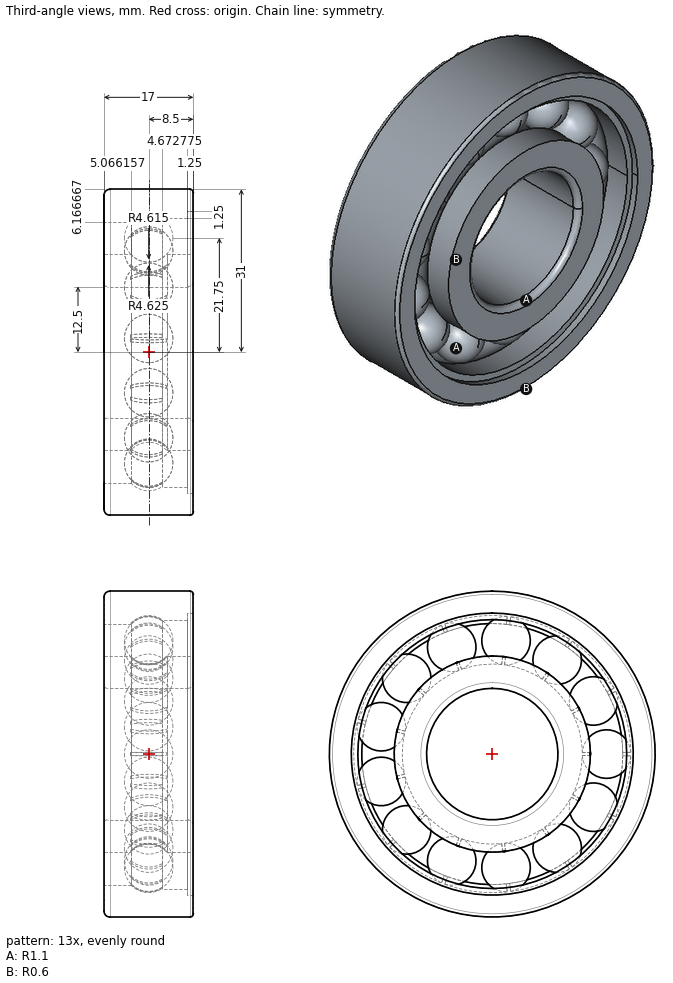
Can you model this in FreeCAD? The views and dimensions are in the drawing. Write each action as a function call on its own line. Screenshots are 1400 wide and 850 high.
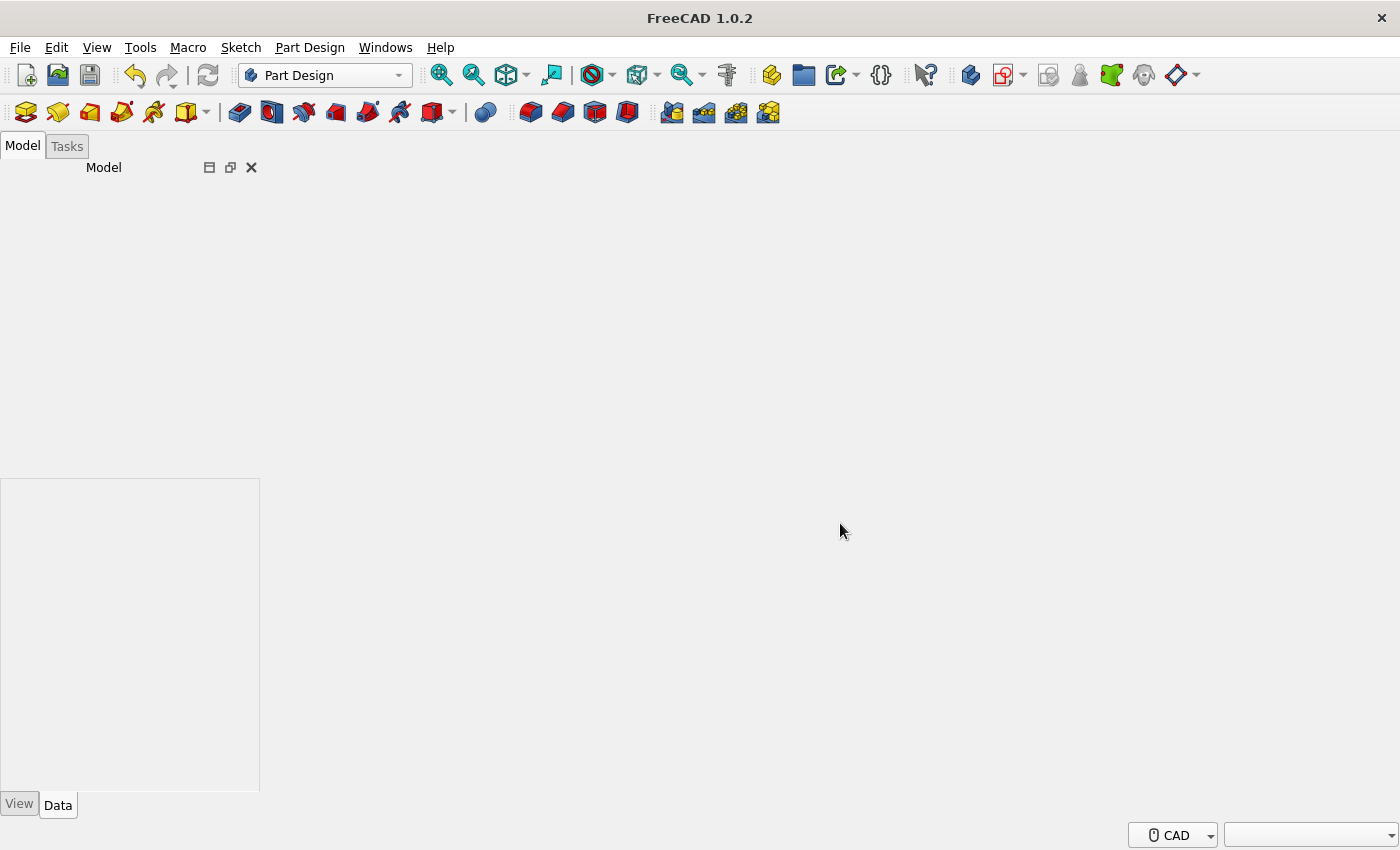
click(26, 76)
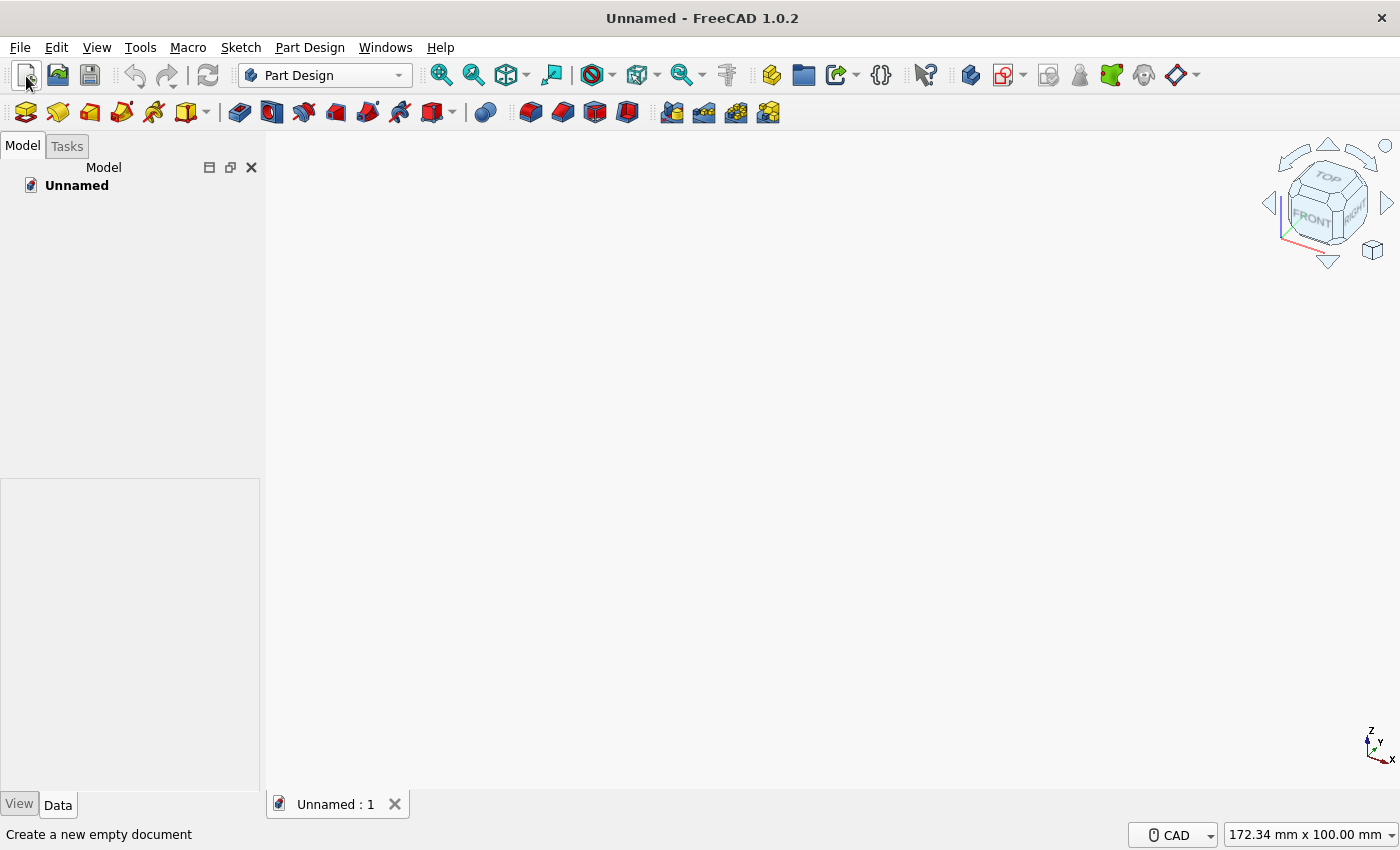
click(1004, 76)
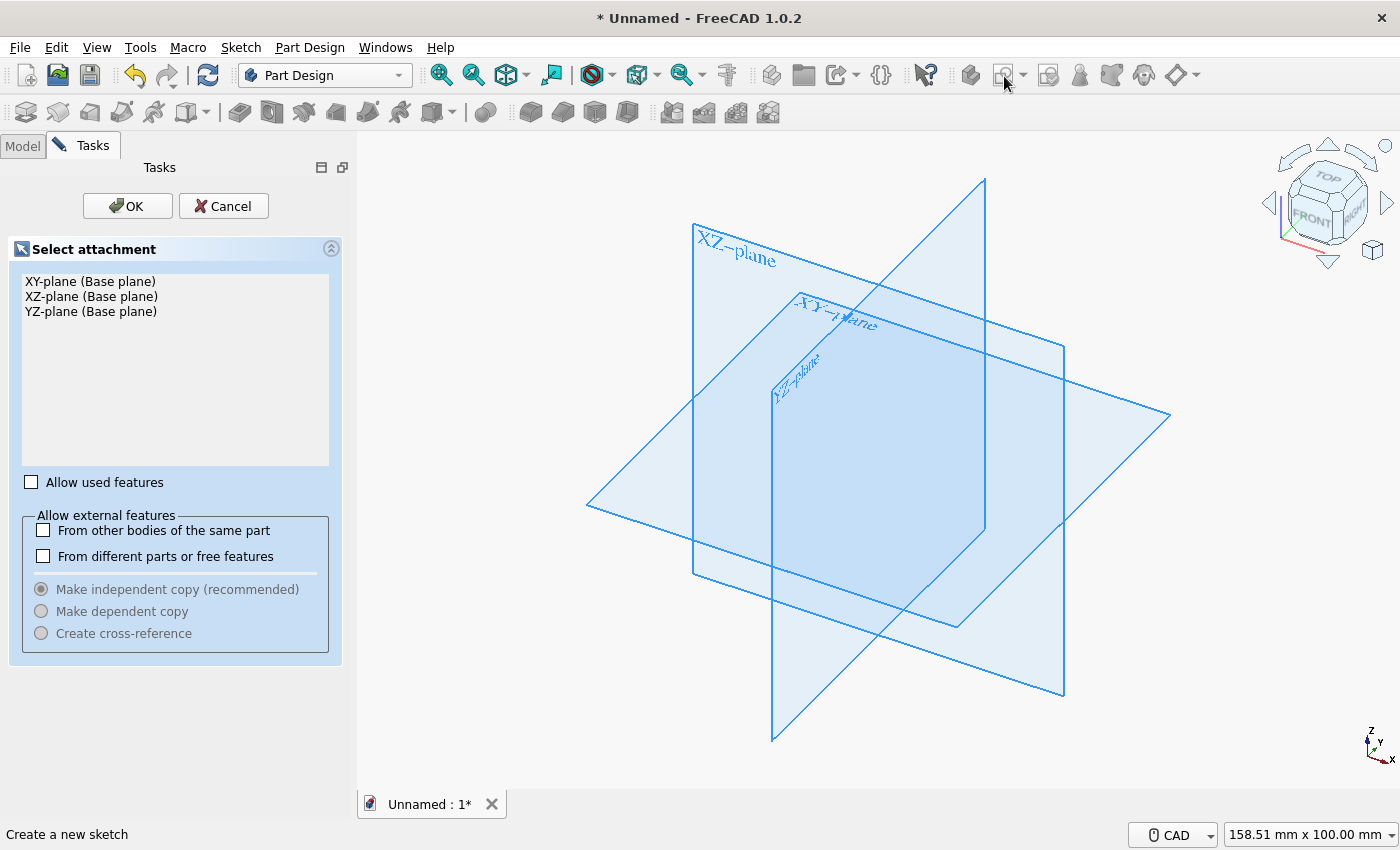
click(82, 282)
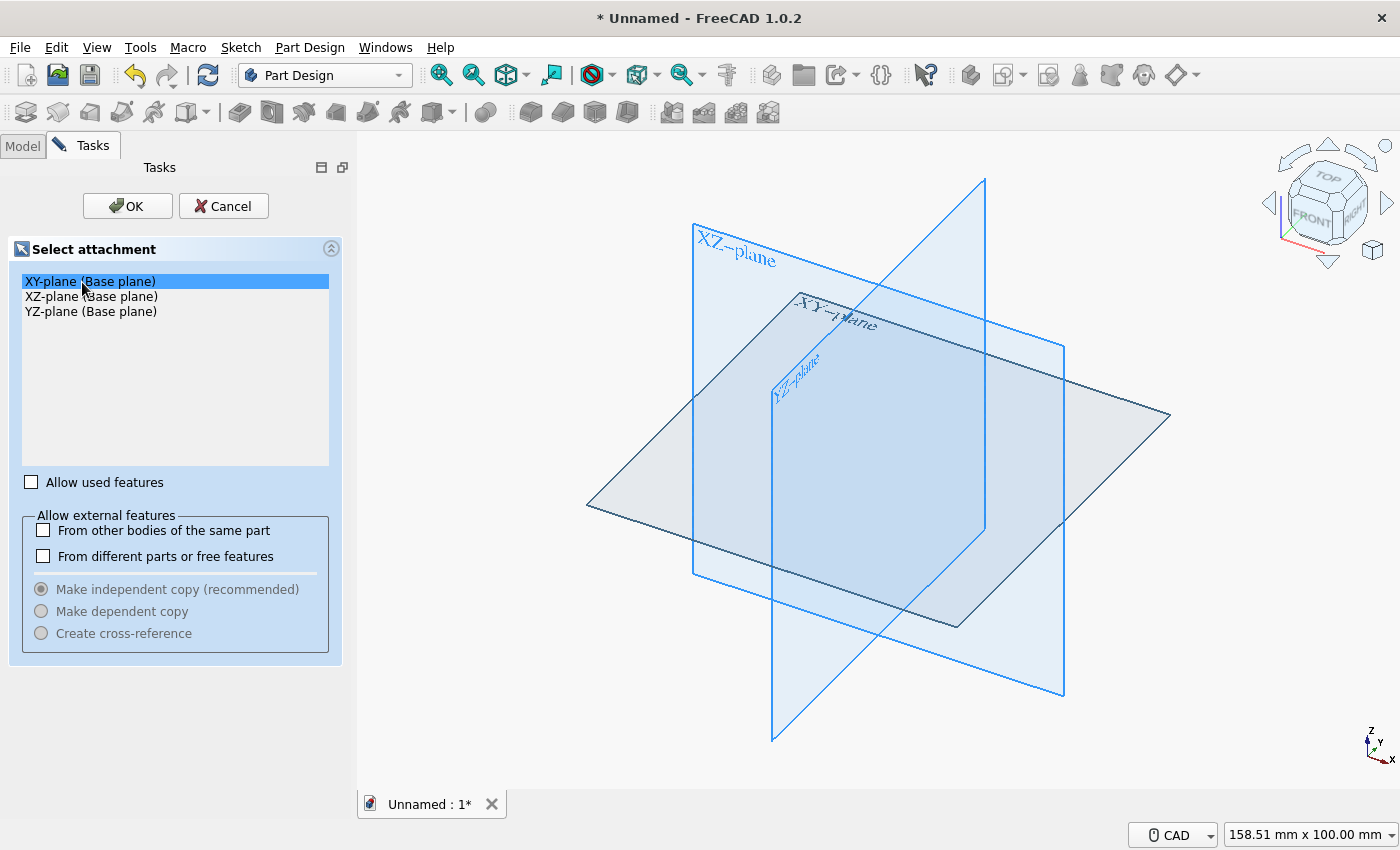
click(128, 206)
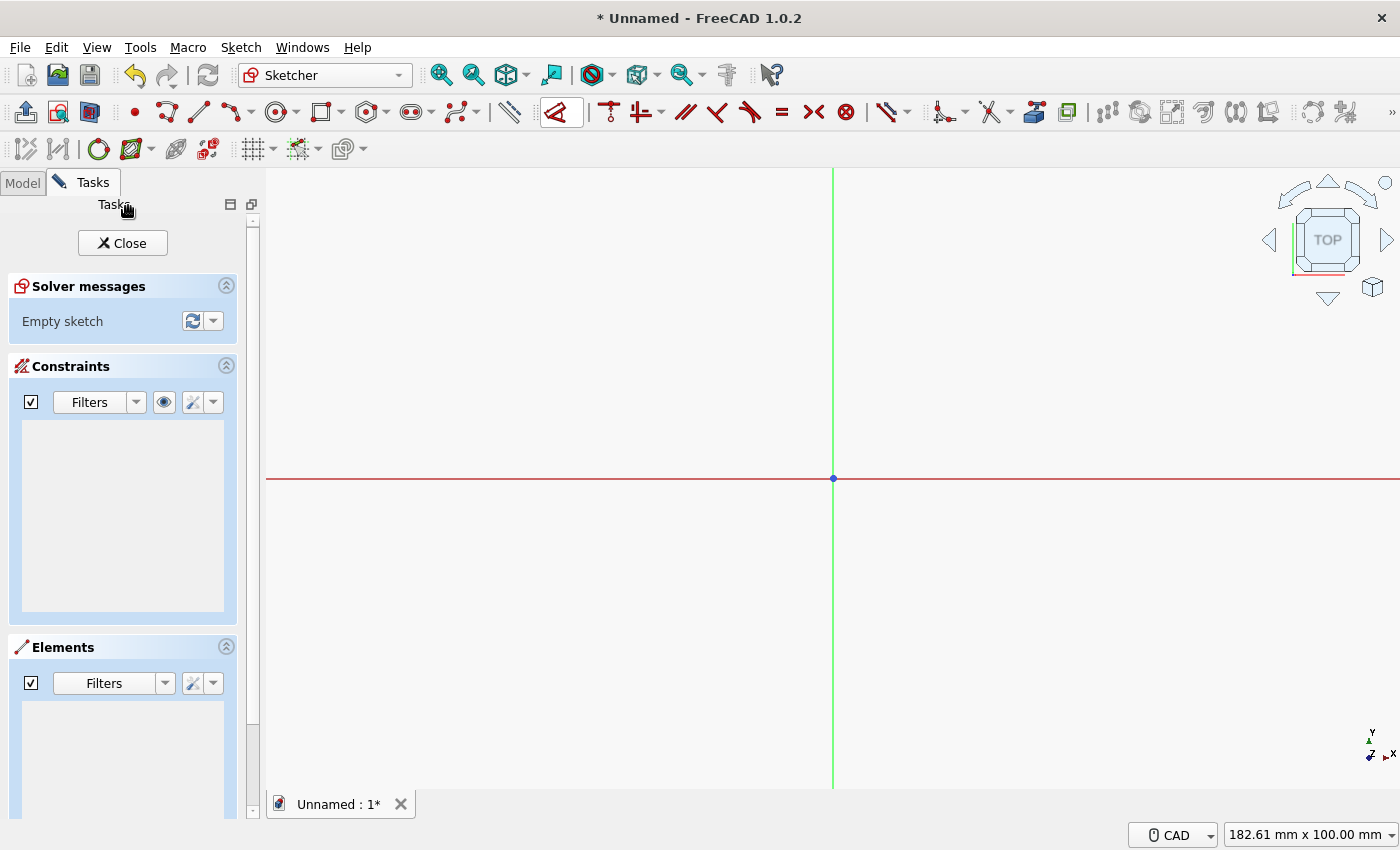
scroll(891, 372, up, 5)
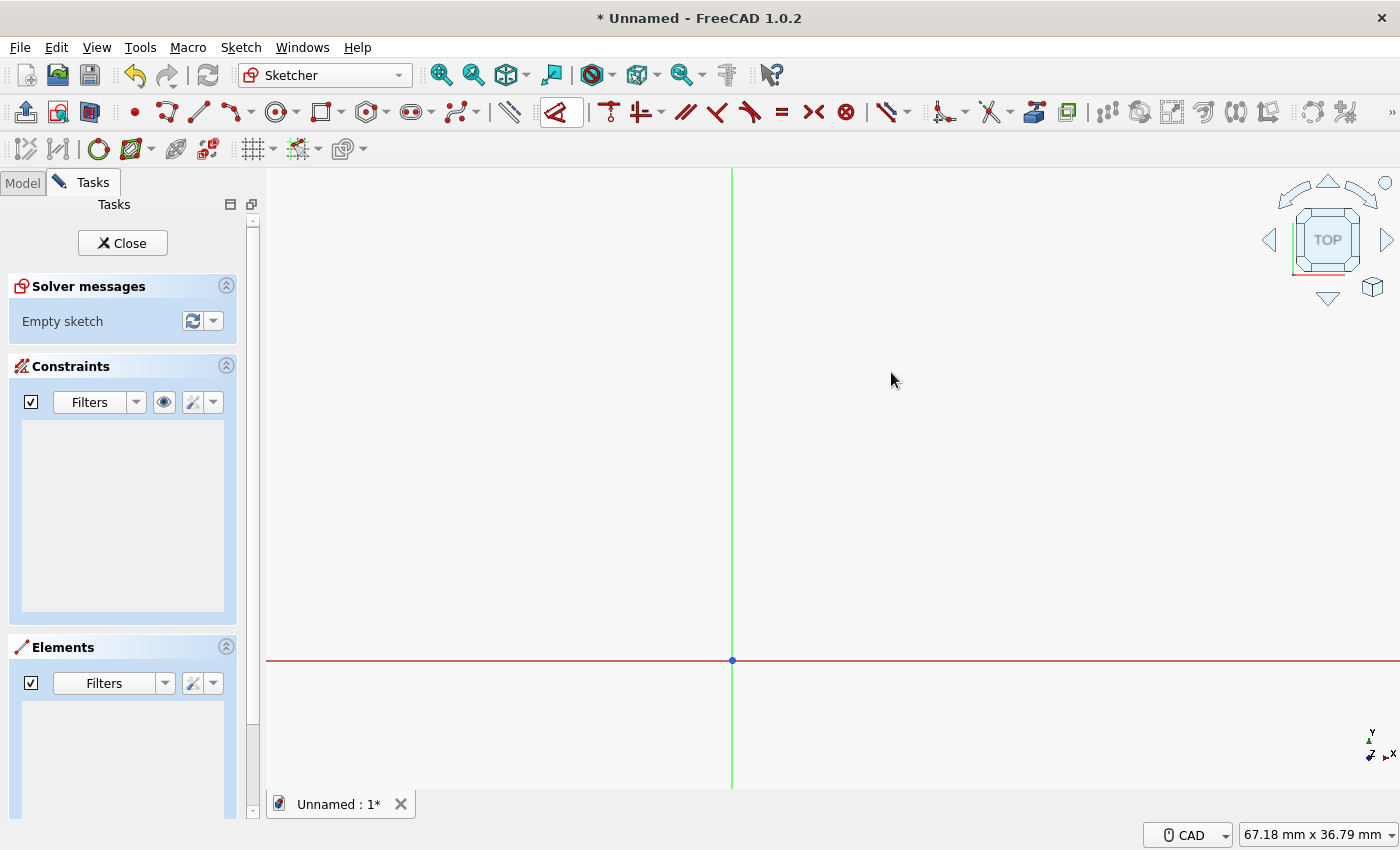
key(g)
key(l)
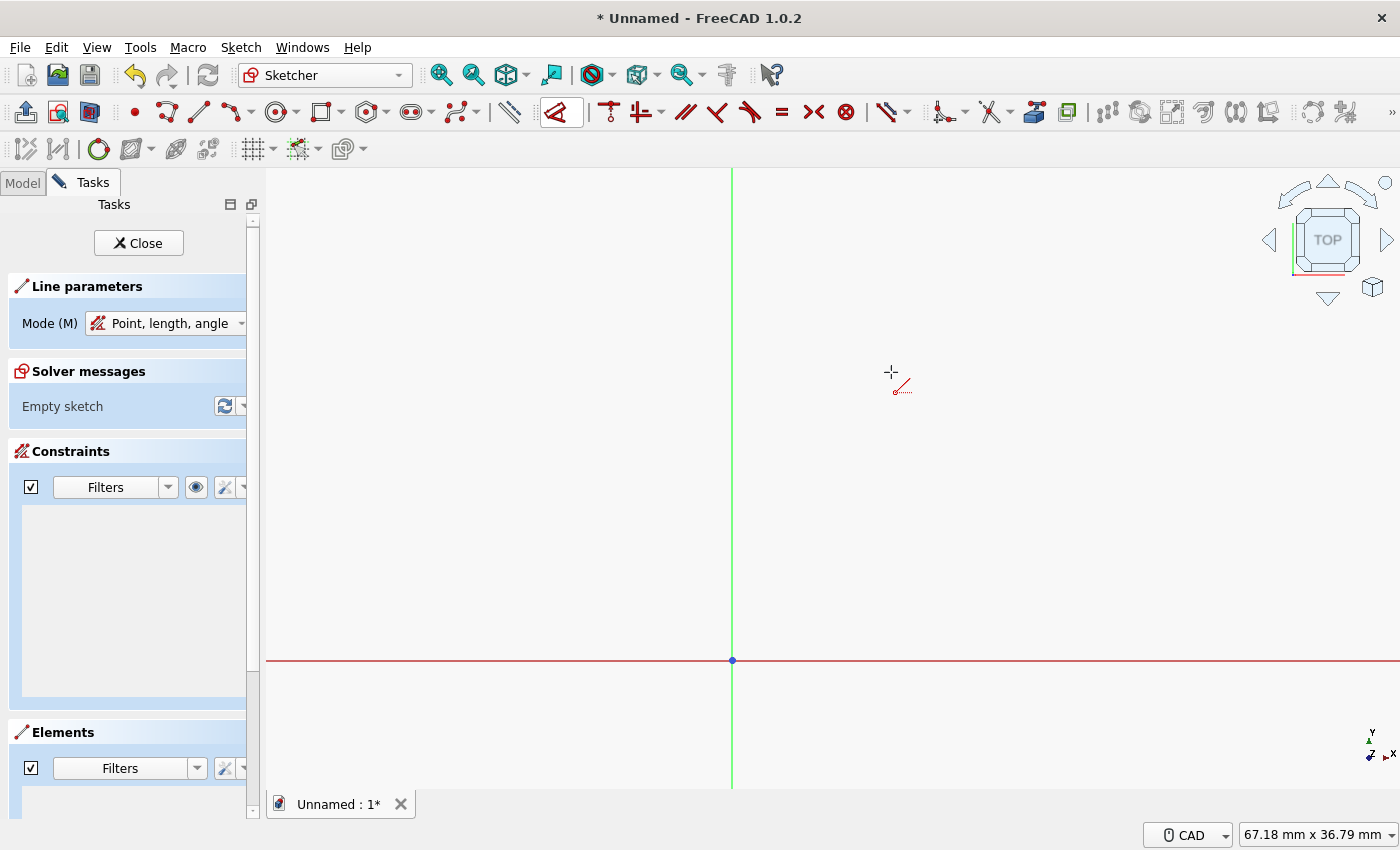
click(810, 294)
click(654, 294)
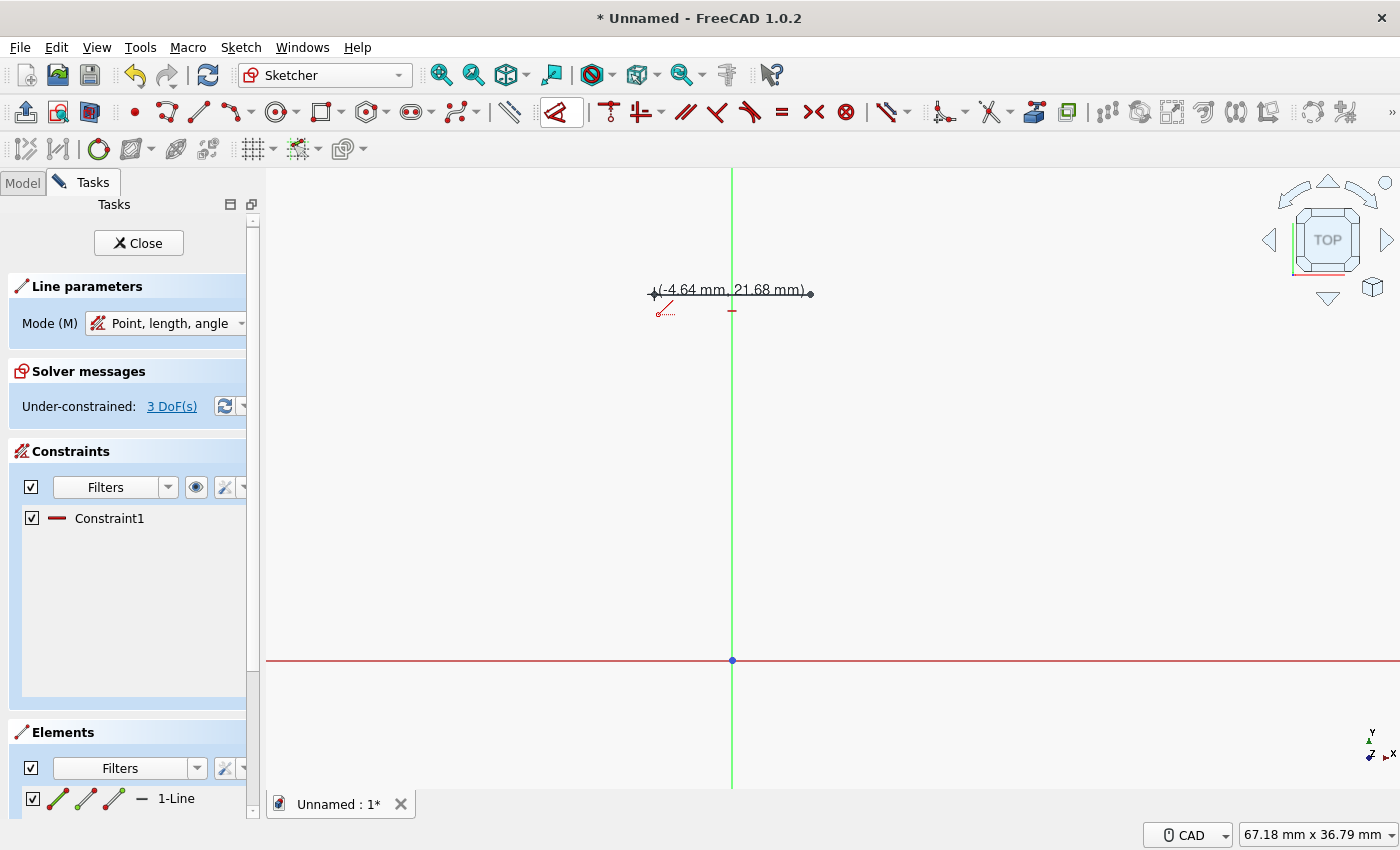
key(g)
key(3)
key(a)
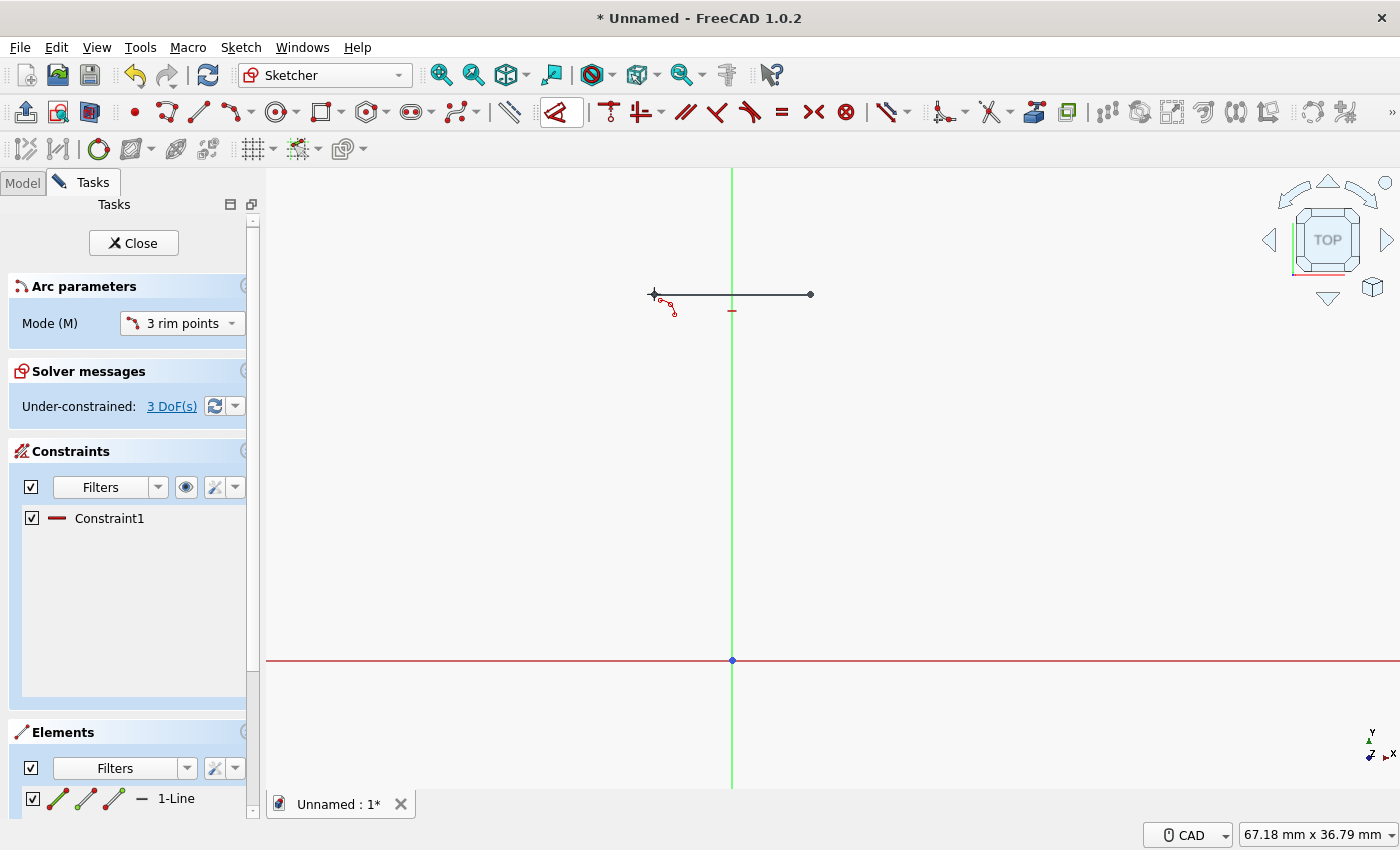
click(654, 295)
click(810, 295)
click(708, 368)